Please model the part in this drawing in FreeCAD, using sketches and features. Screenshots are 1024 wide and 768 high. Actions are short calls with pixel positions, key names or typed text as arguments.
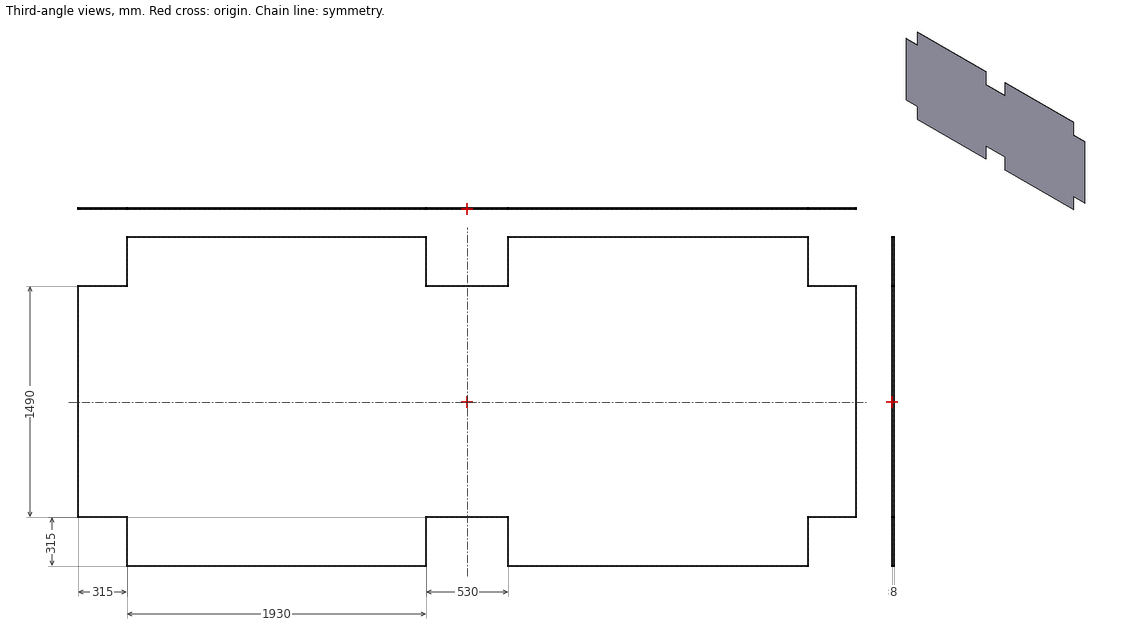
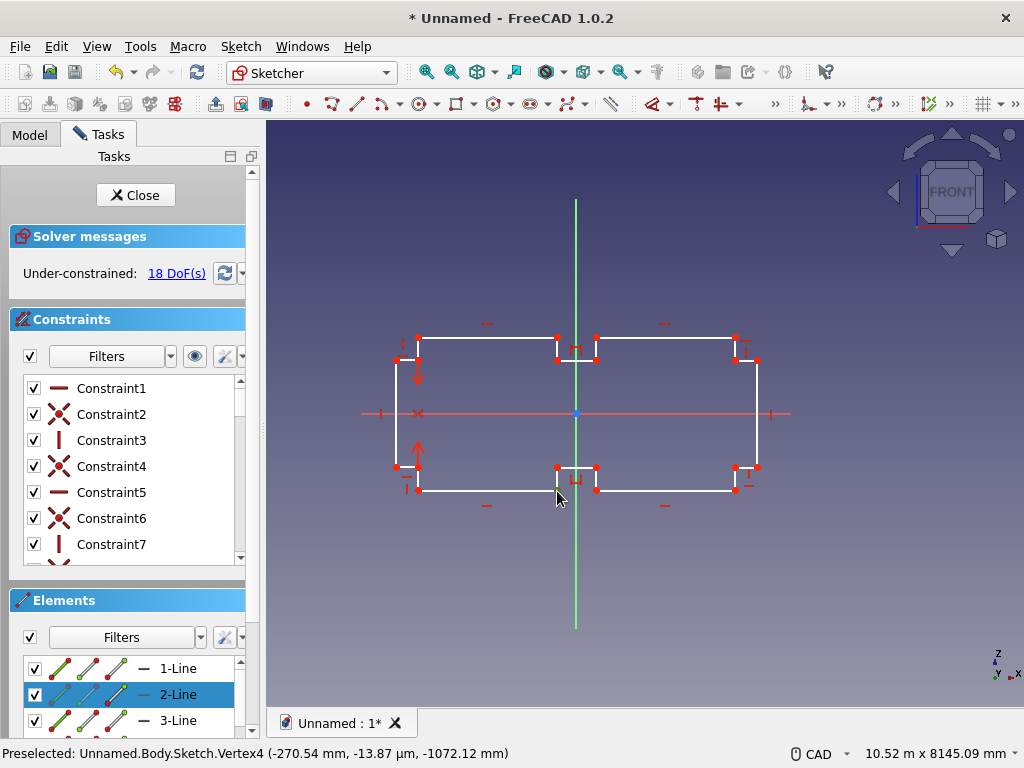
click(557, 338)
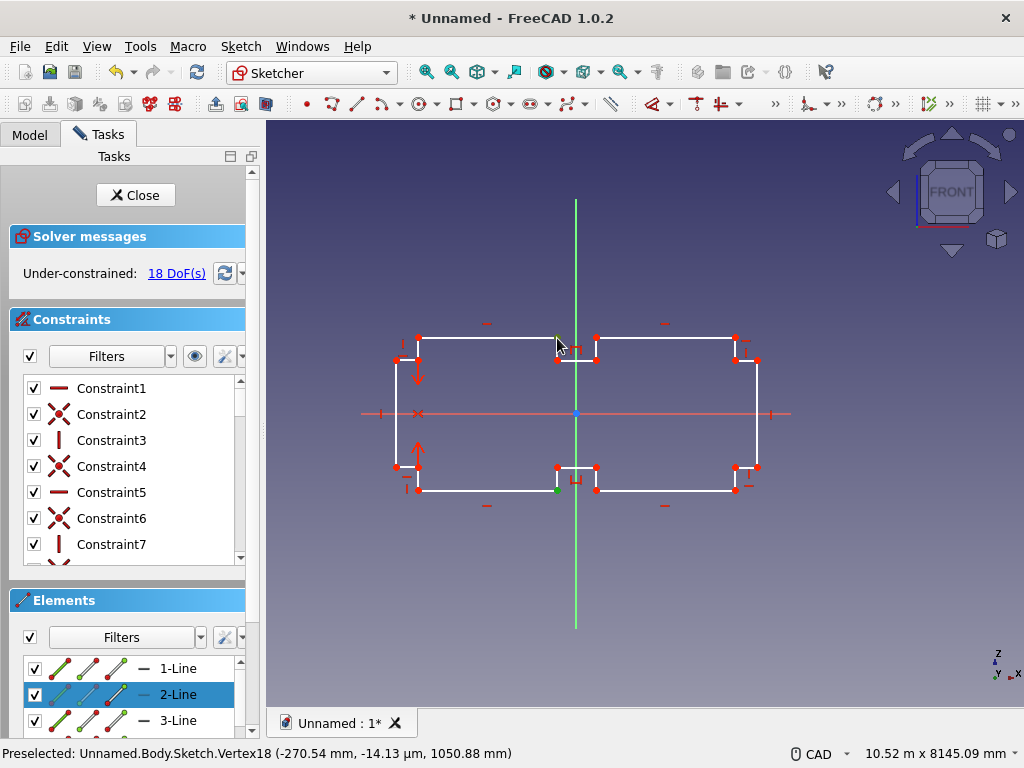
click(455, 414)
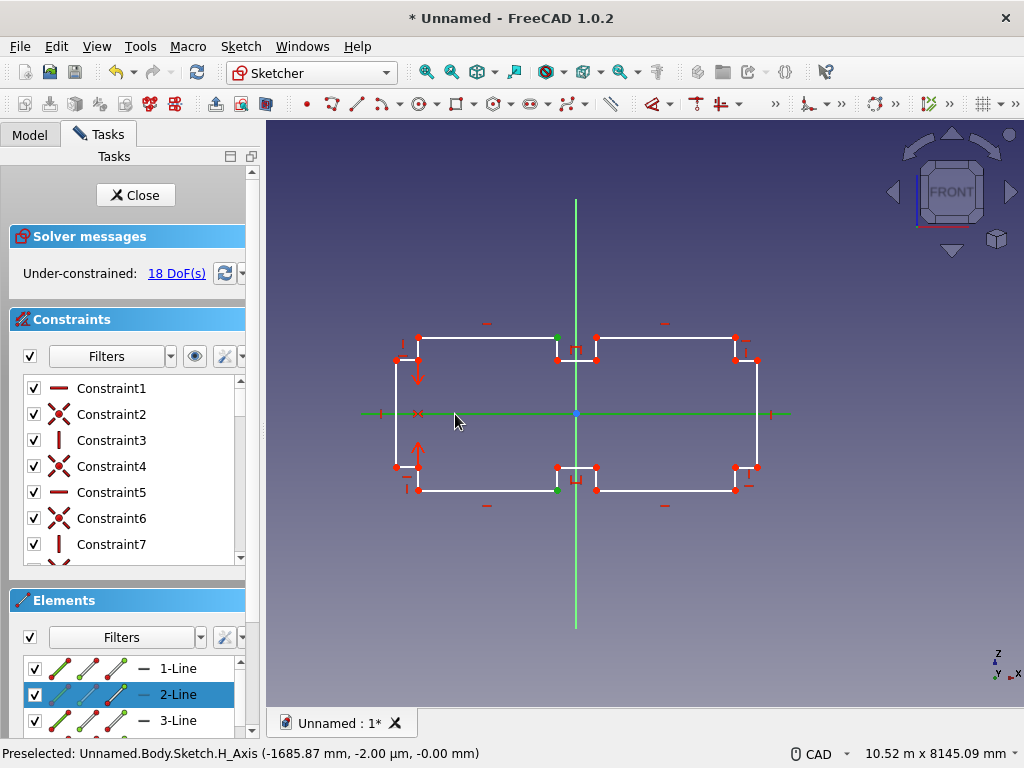
key(s)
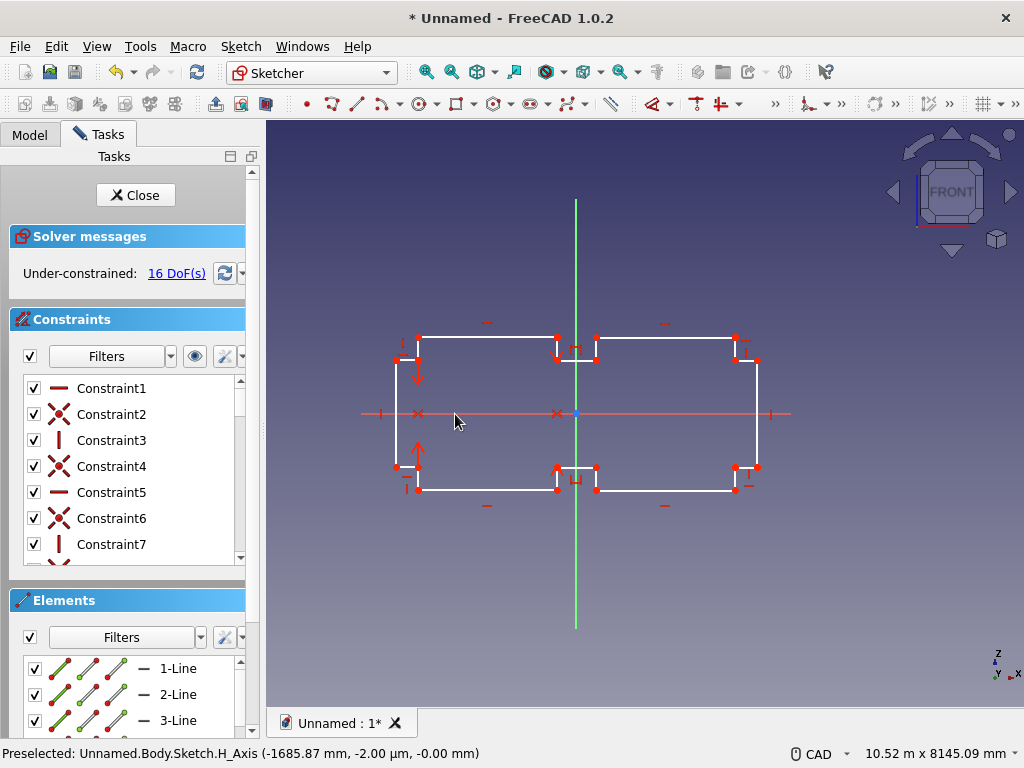
click(596, 468)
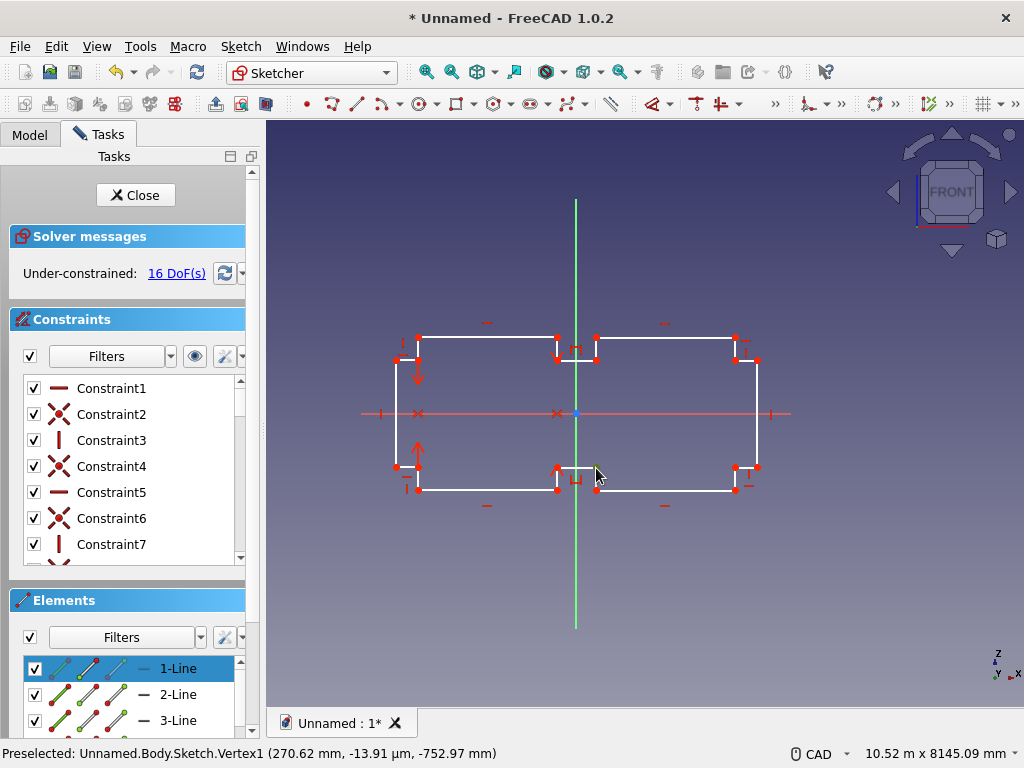
click(596, 361)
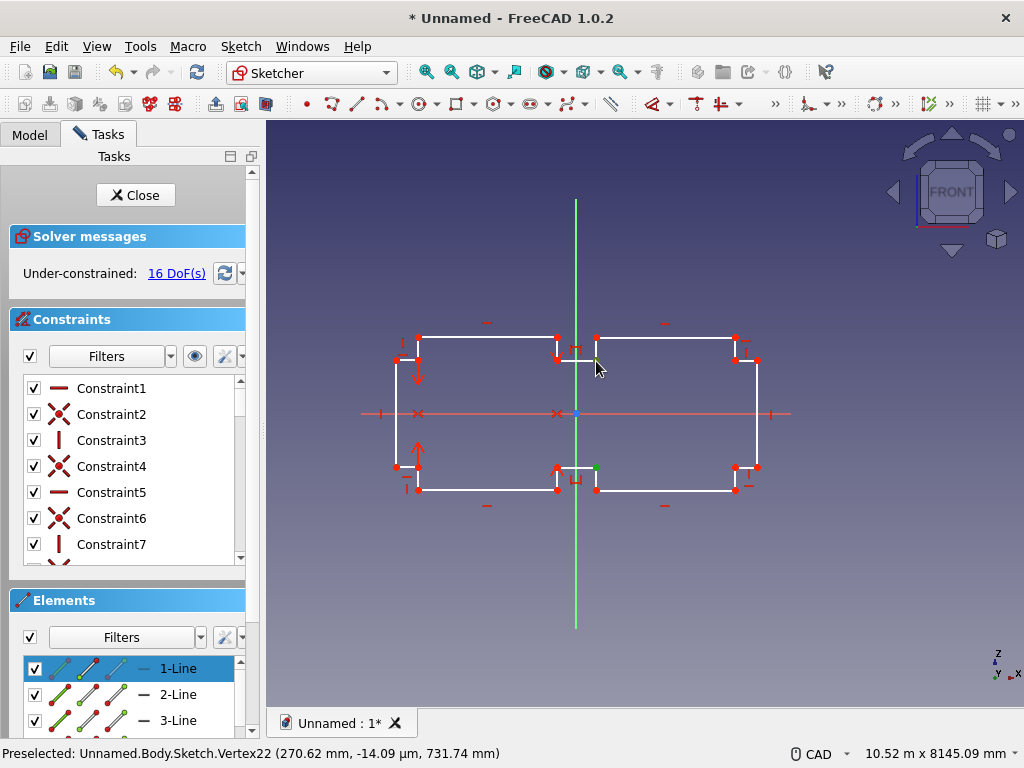
click(455, 414)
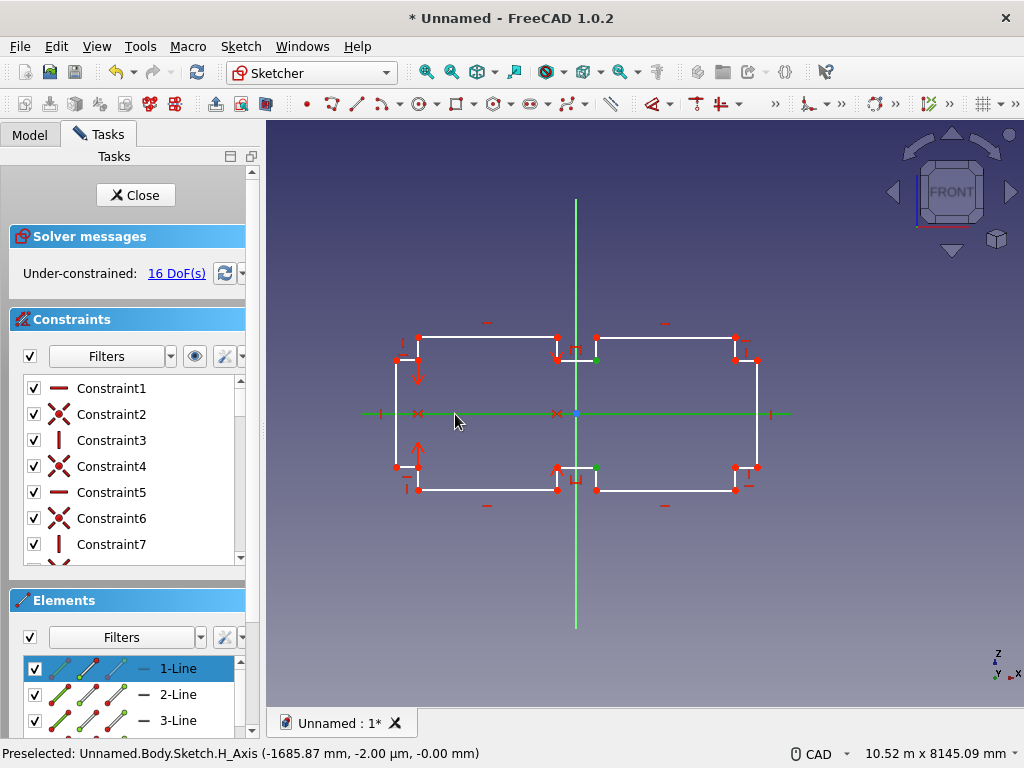
key(s)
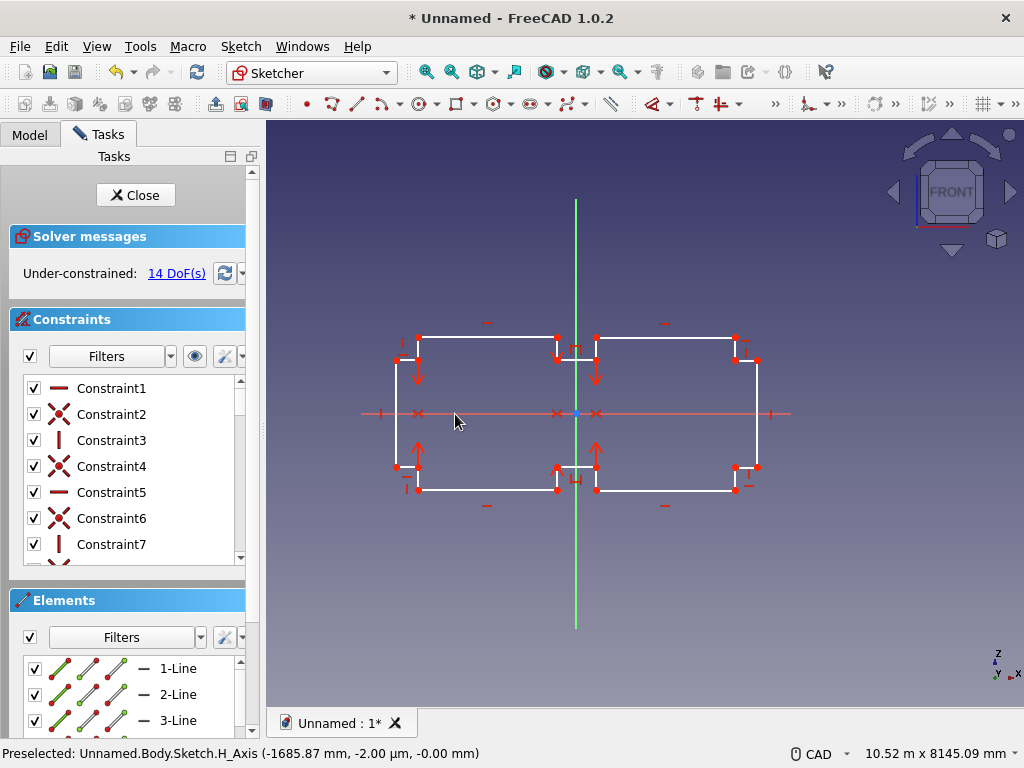
click(557, 337)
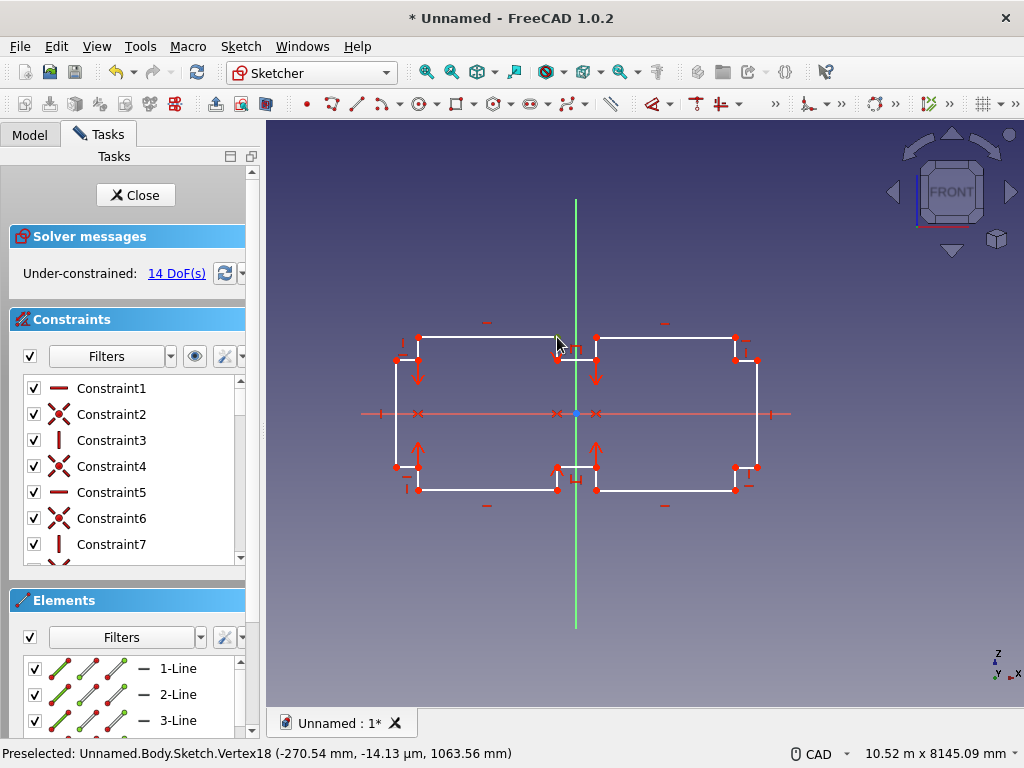
click(596, 338)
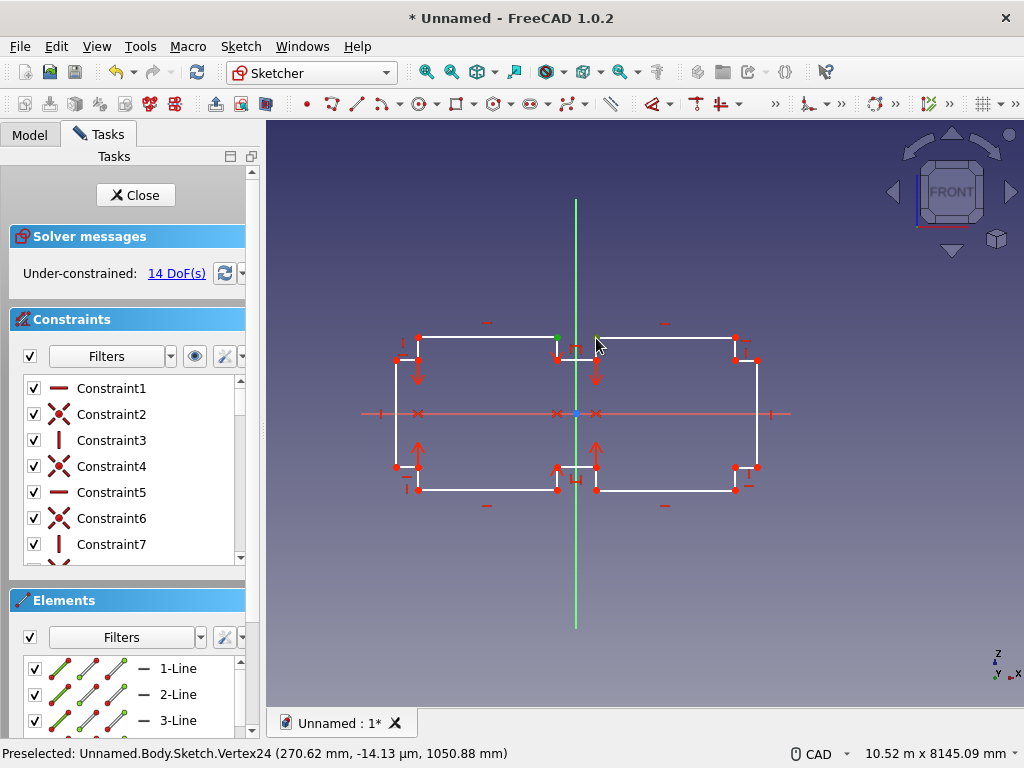
click(576, 603)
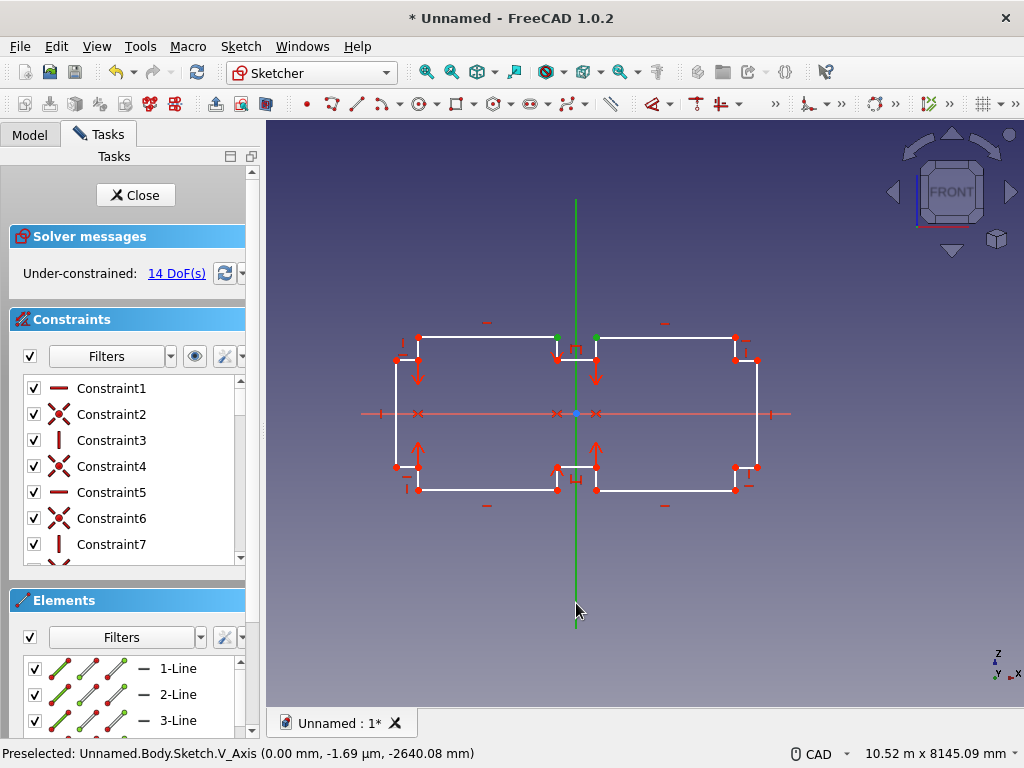
key(s)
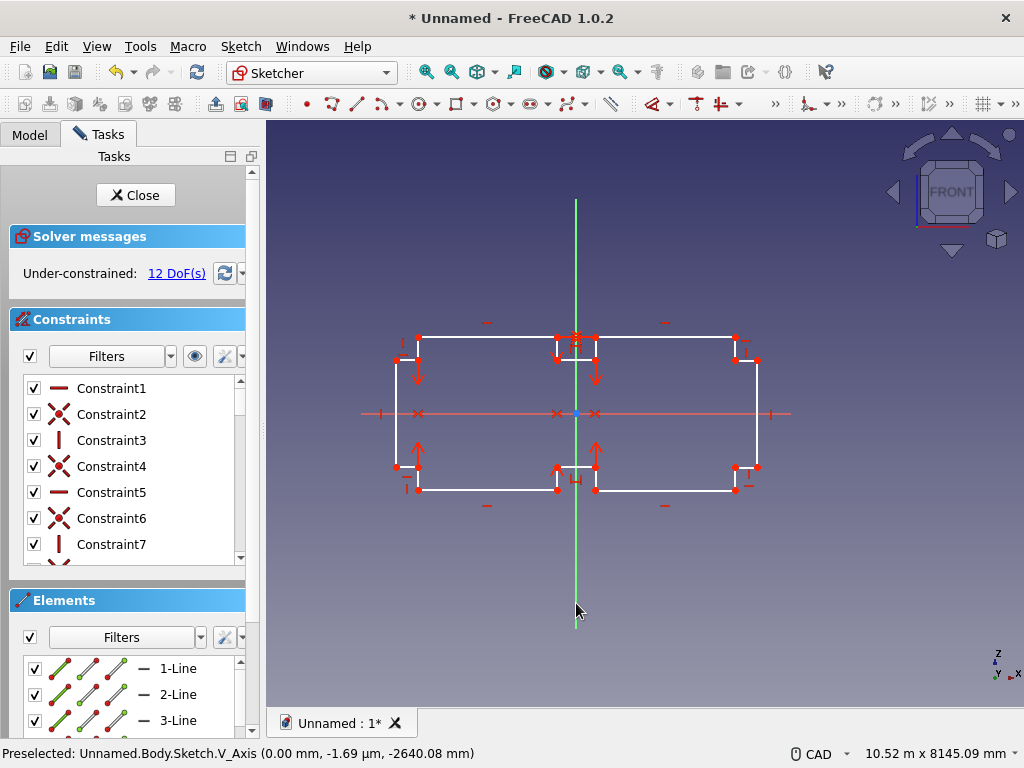
click(418, 360)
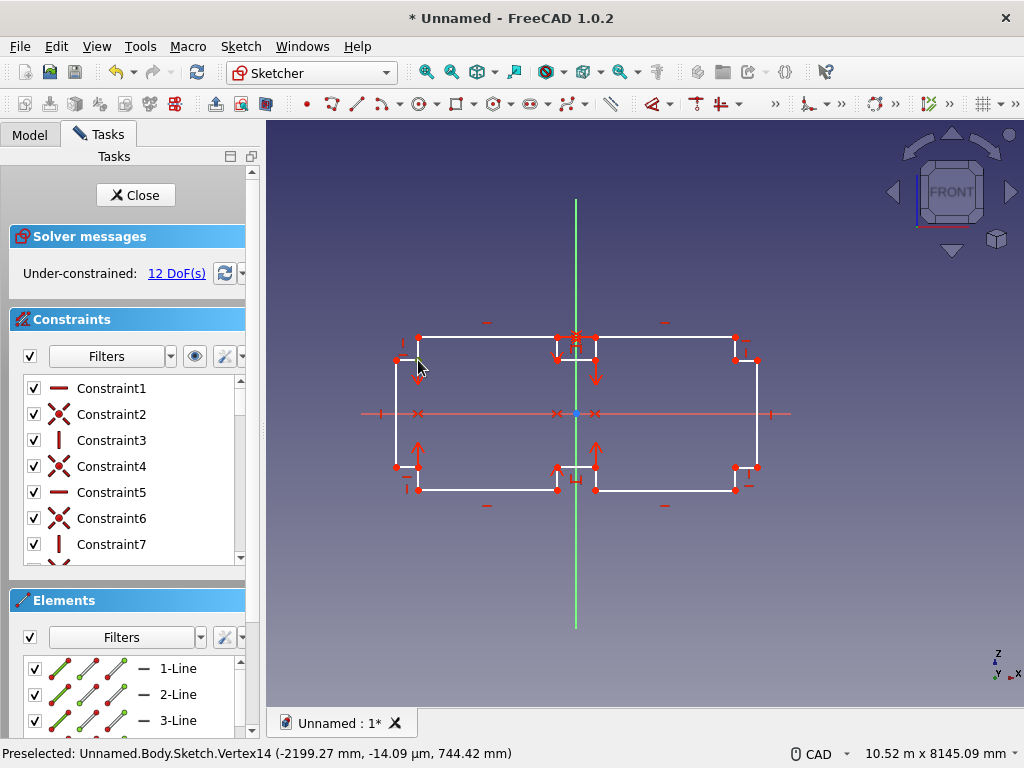
click(735, 361)